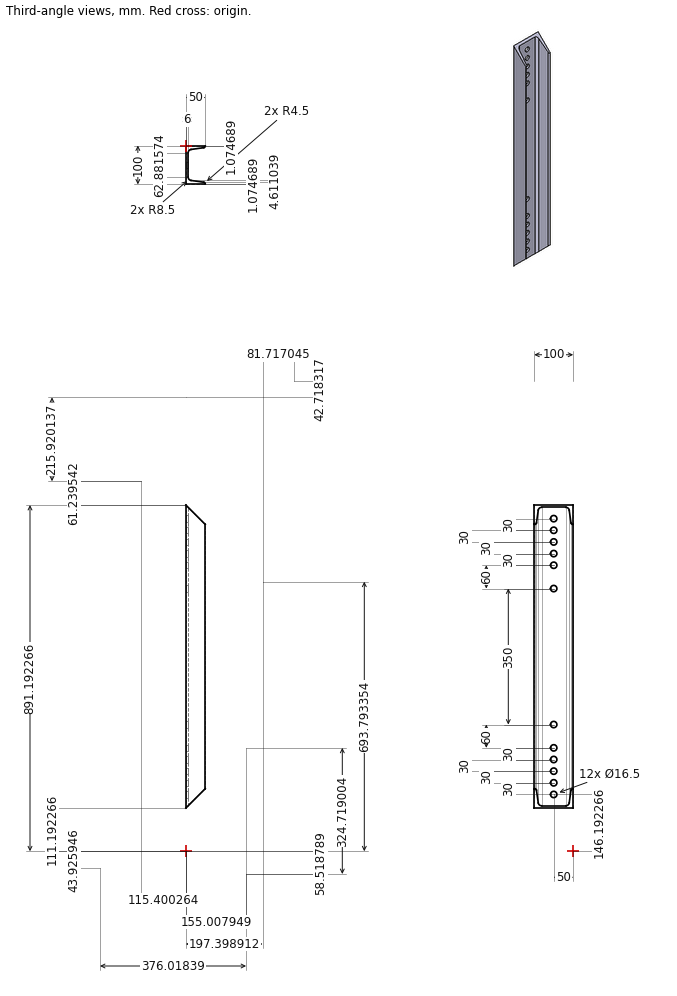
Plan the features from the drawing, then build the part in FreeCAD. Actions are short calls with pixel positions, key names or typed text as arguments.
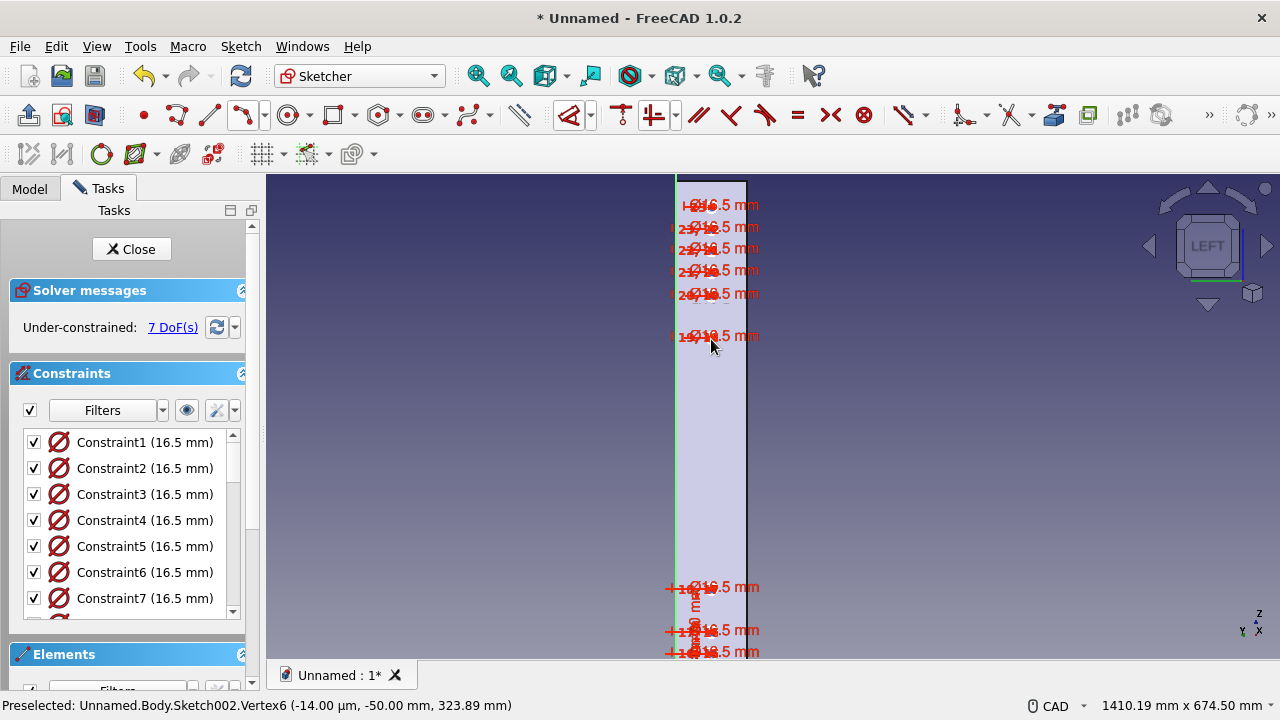
click(711, 338)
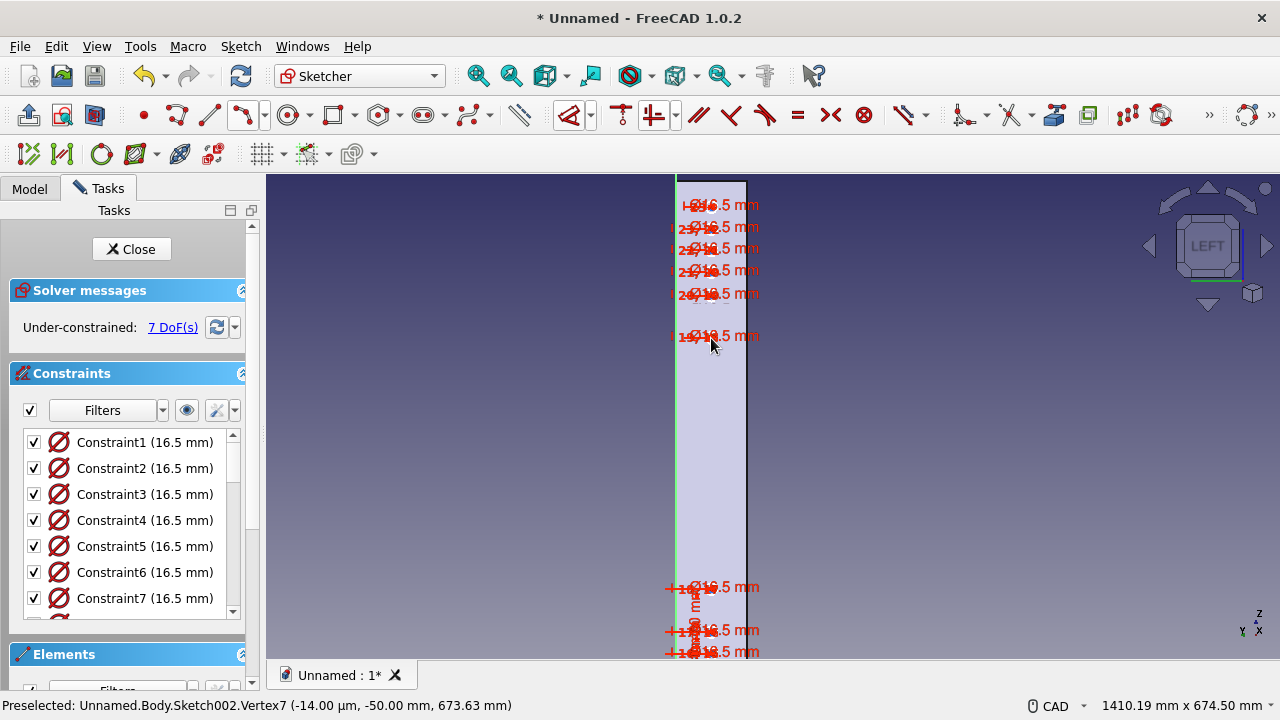
click(711, 296)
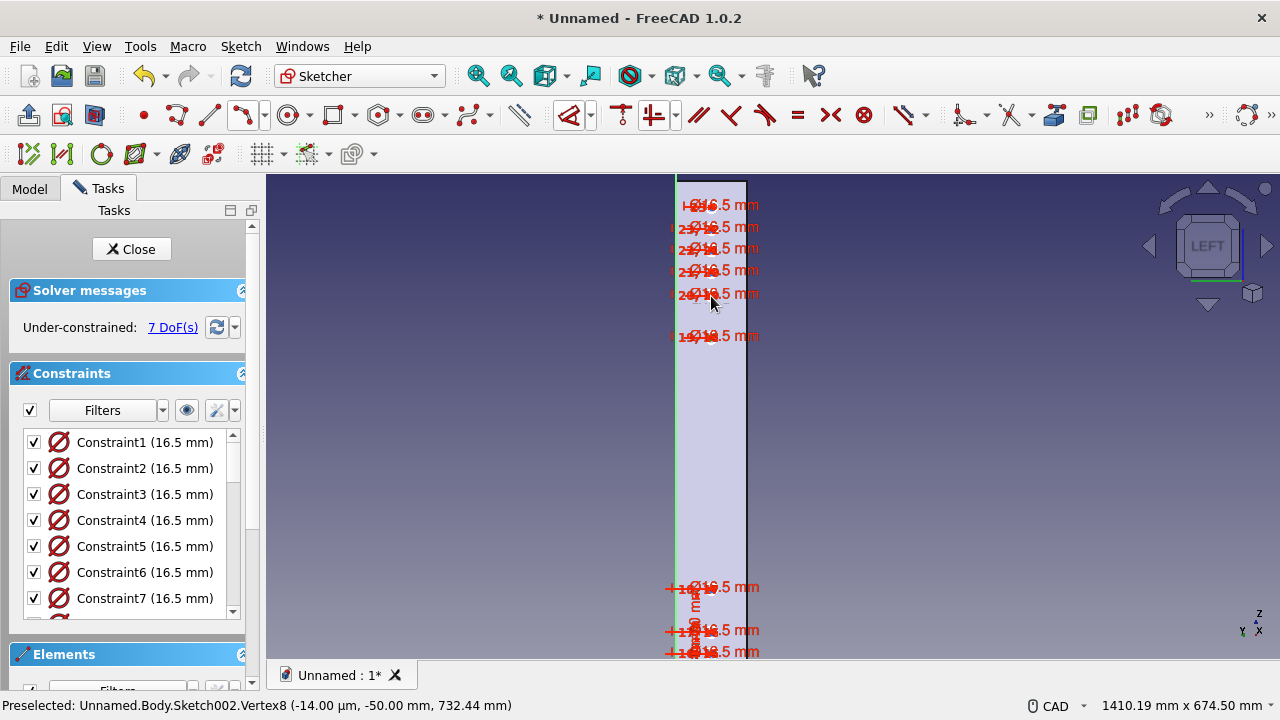
click(590, 116)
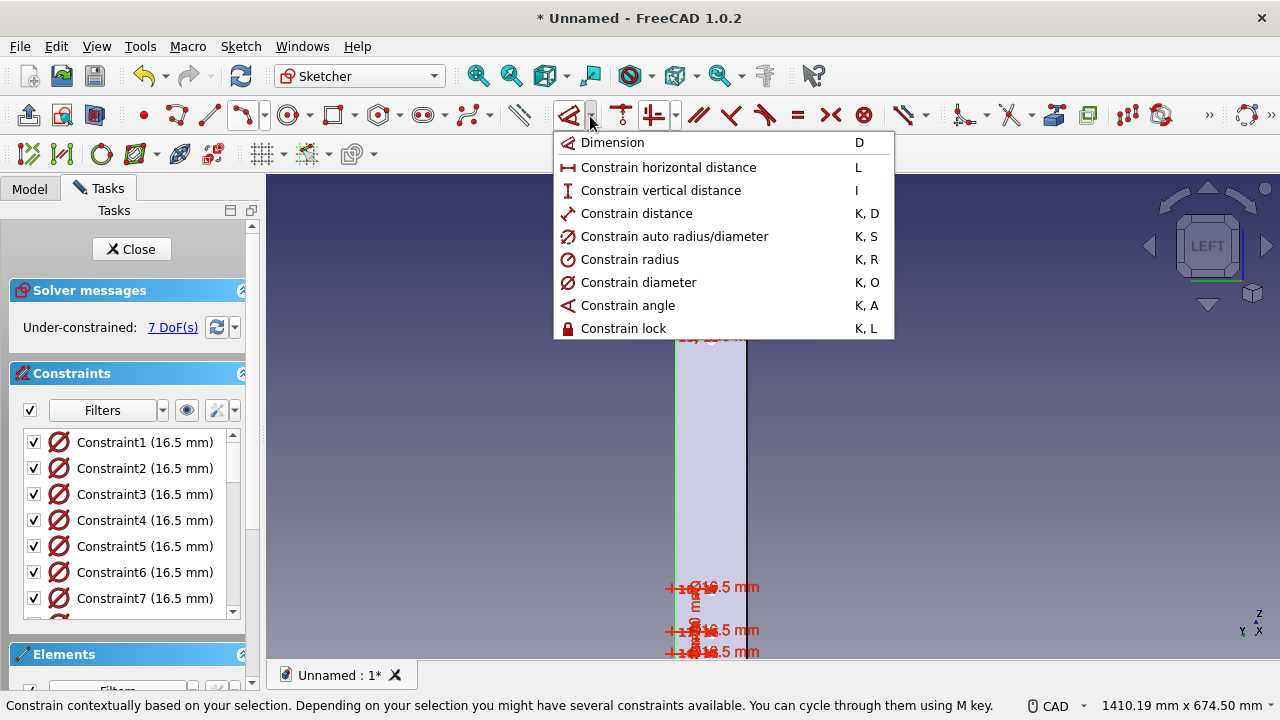
click(724, 190)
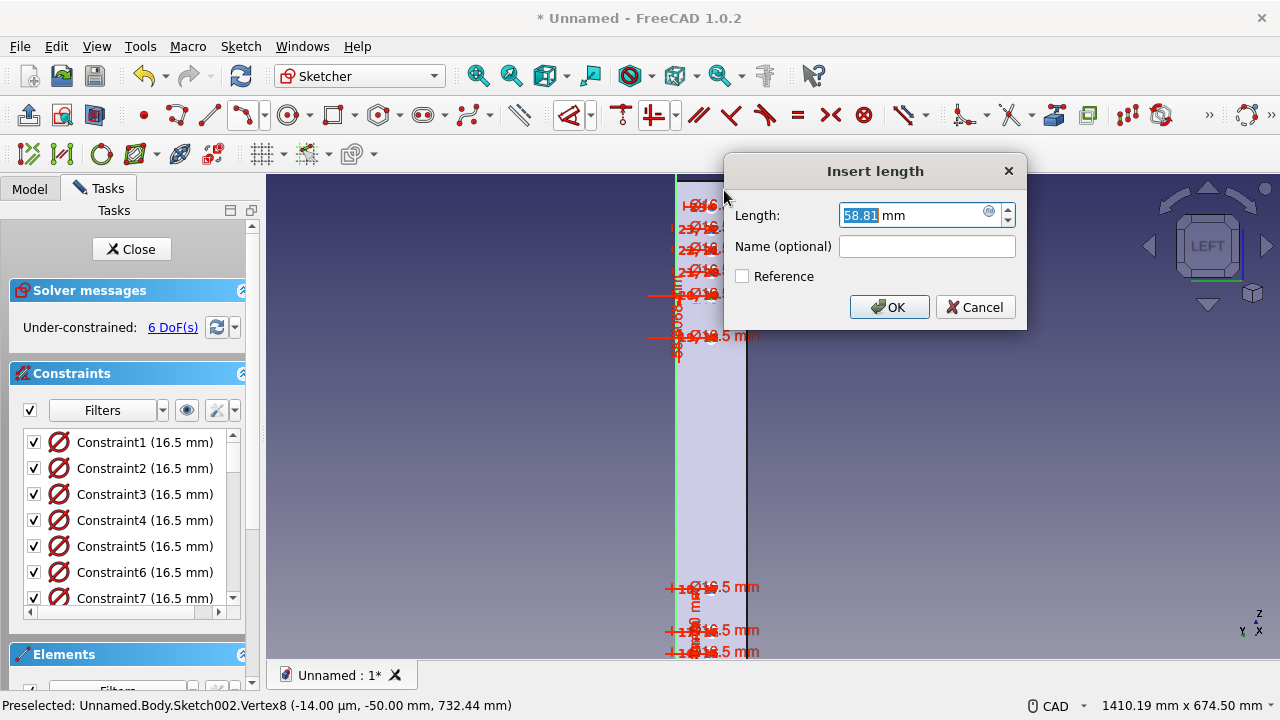
text(60)
key(Return)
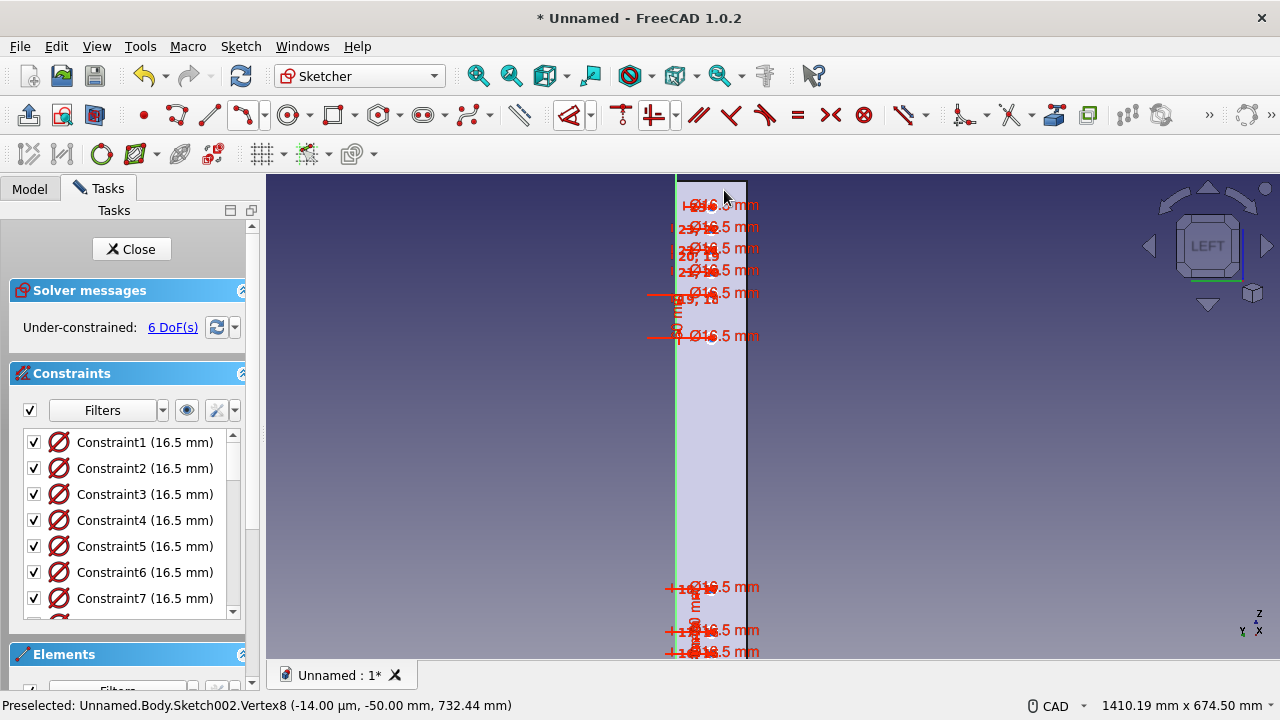
scroll(711, 295, up, 4)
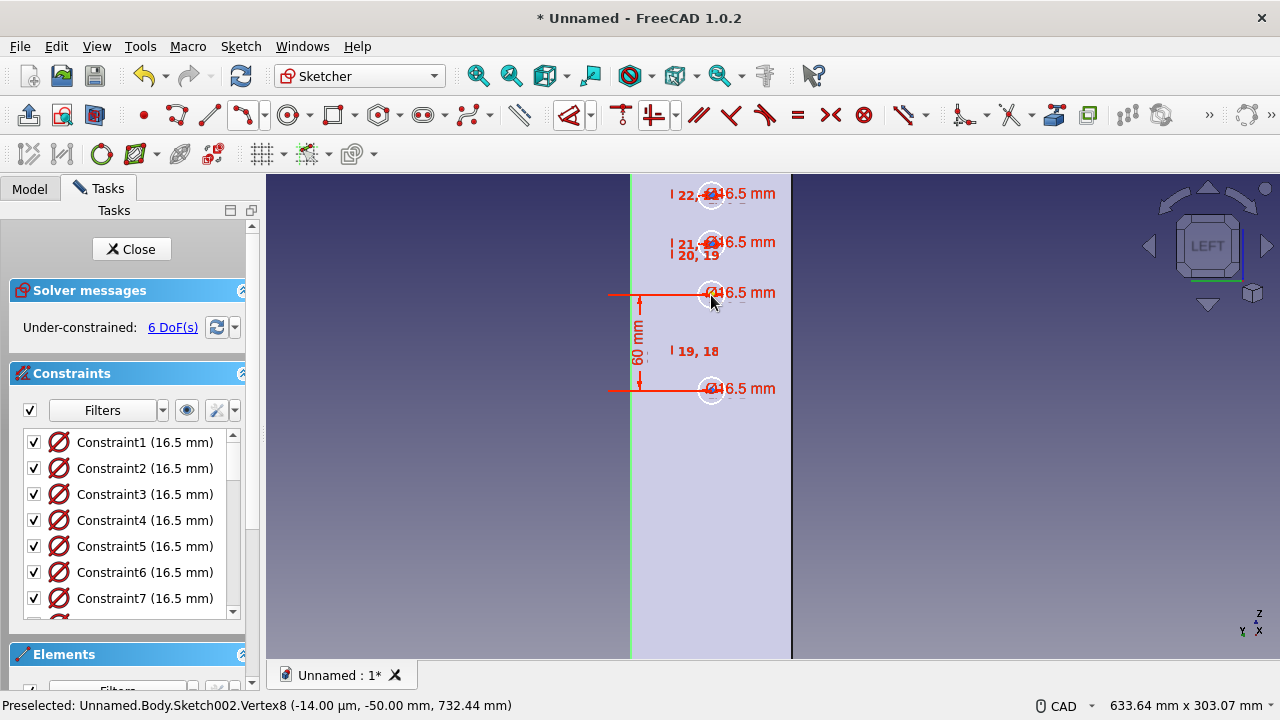
click(712, 295)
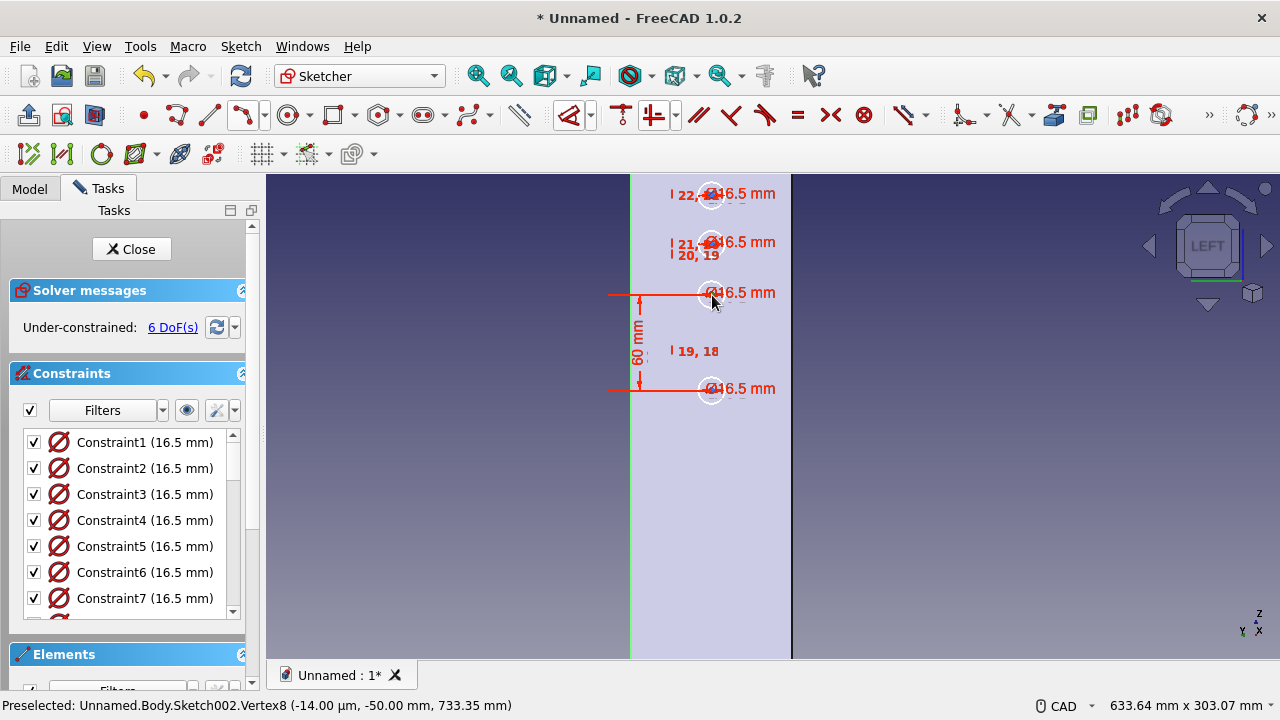
click(712, 244)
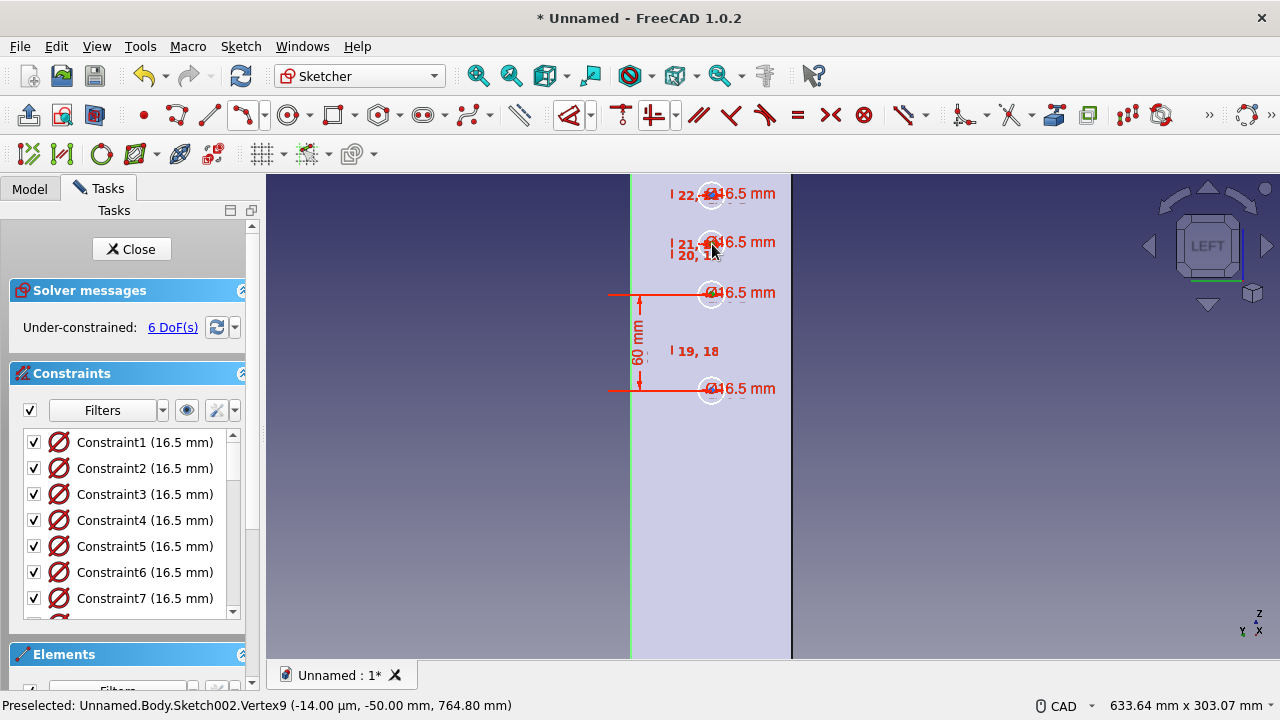
key(i)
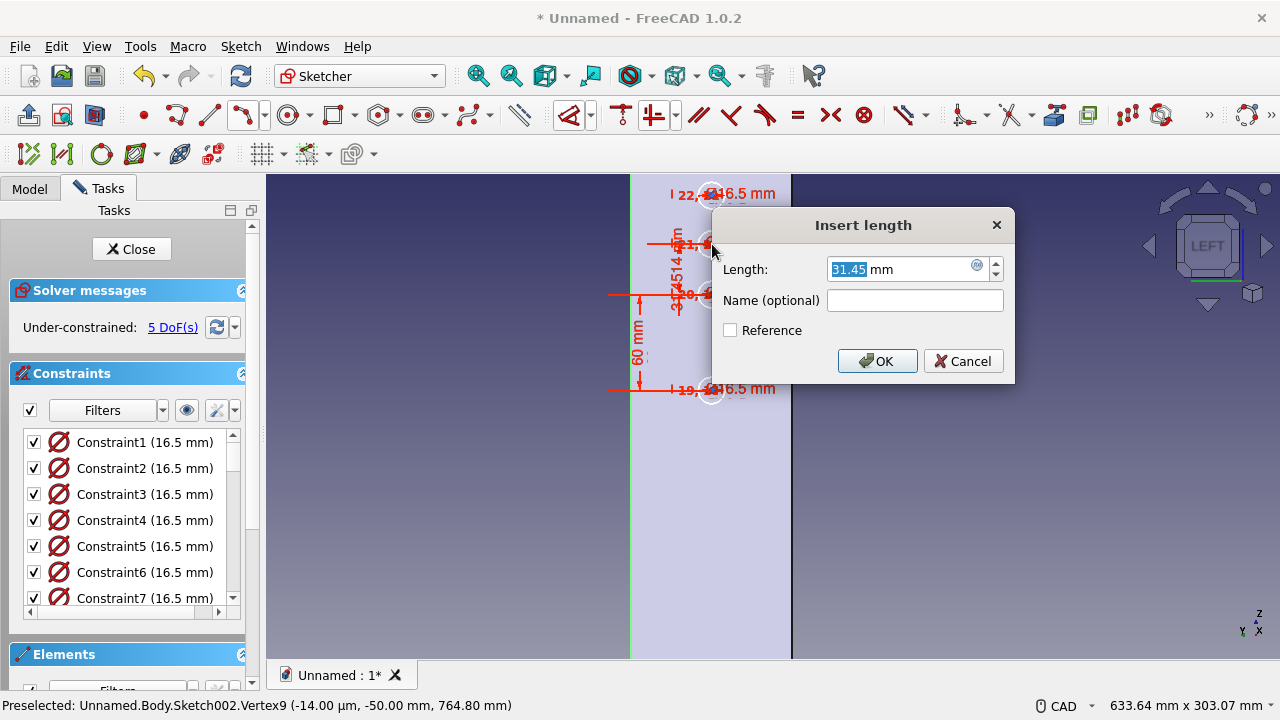
text(30)
key(Return)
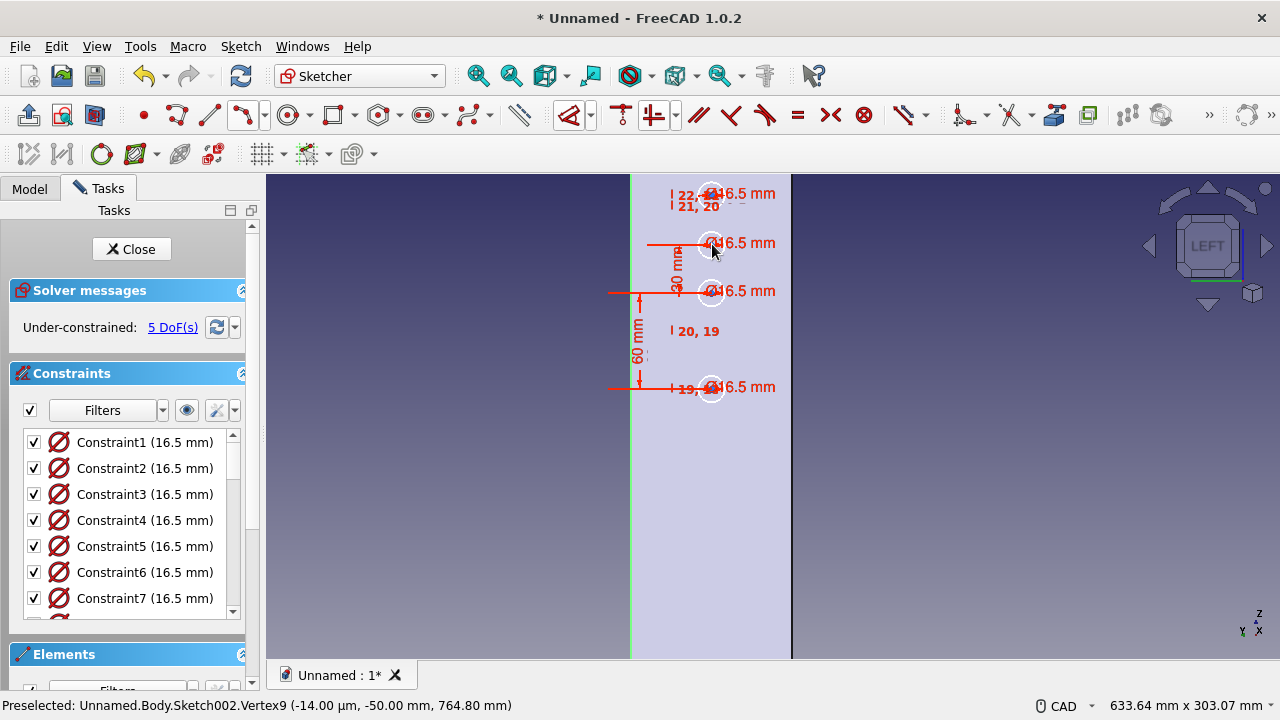
click(712, 245)